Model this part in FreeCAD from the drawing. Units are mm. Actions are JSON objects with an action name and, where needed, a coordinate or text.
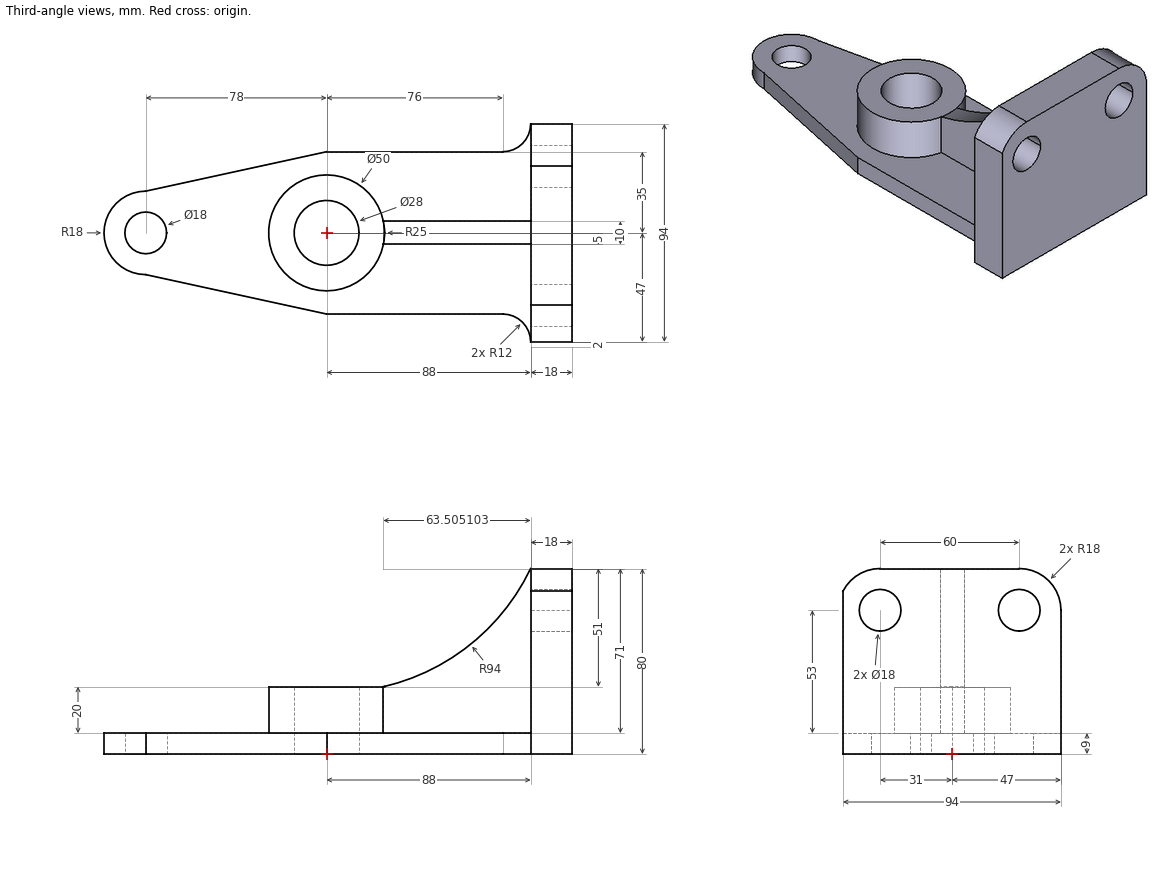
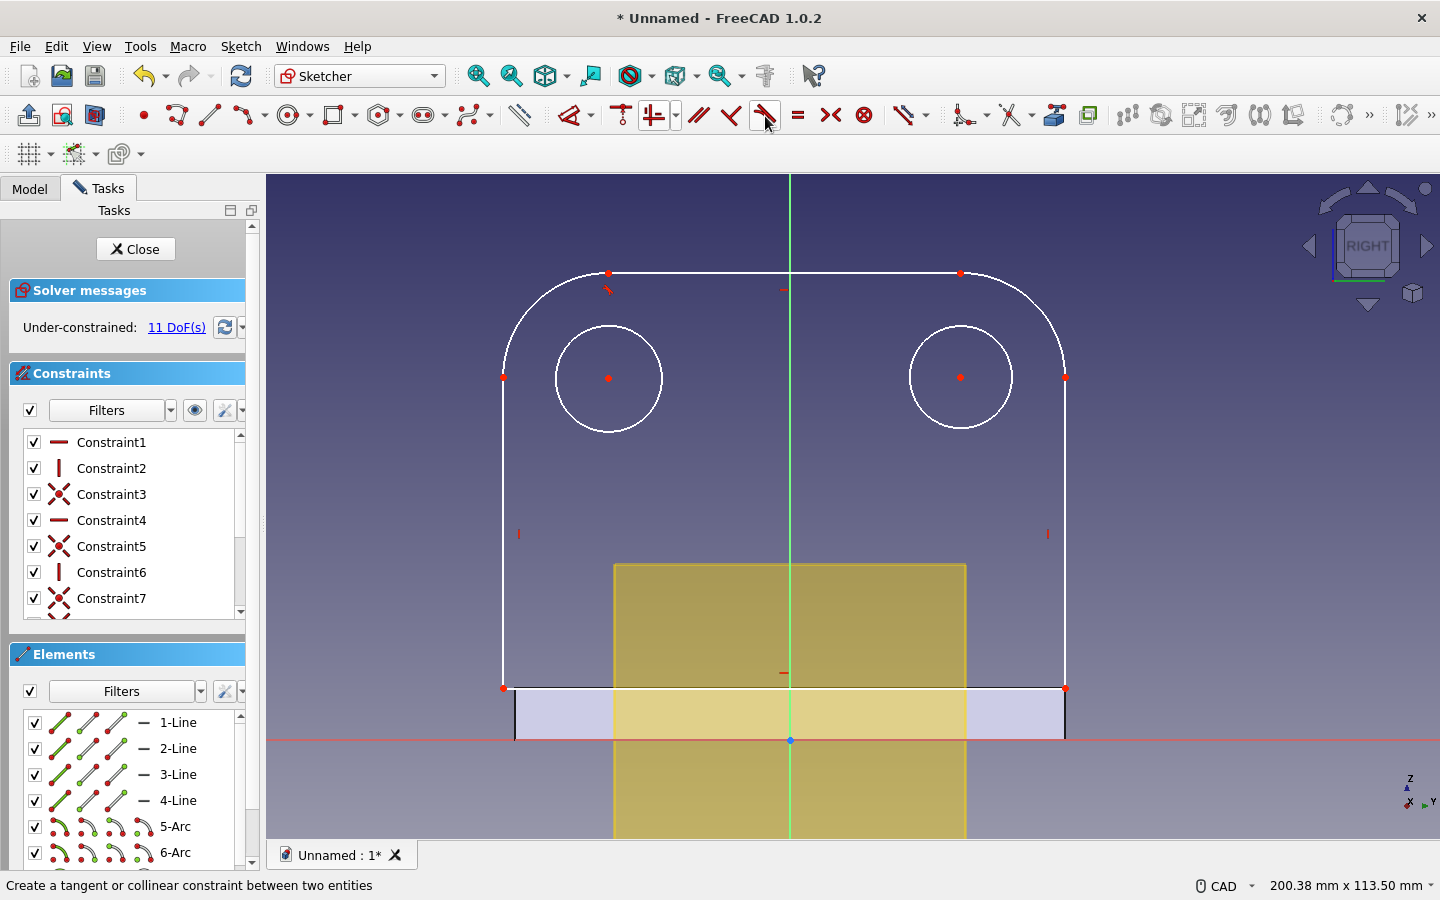
{"action": "left_click", "coordinate": [855, 273]}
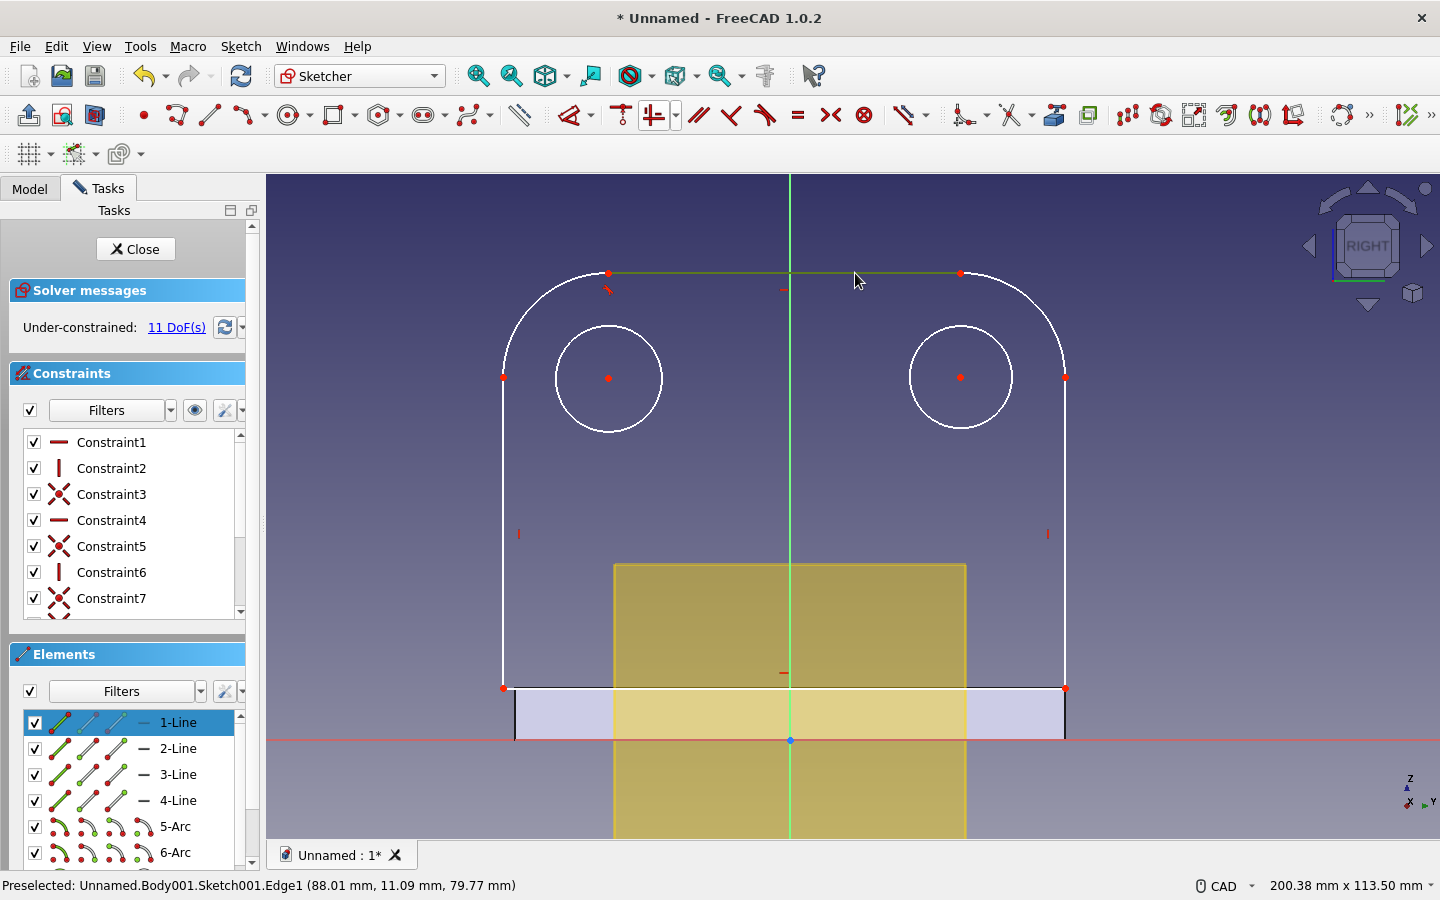
{"action": "left_click", "coordinate": [1054, 330]}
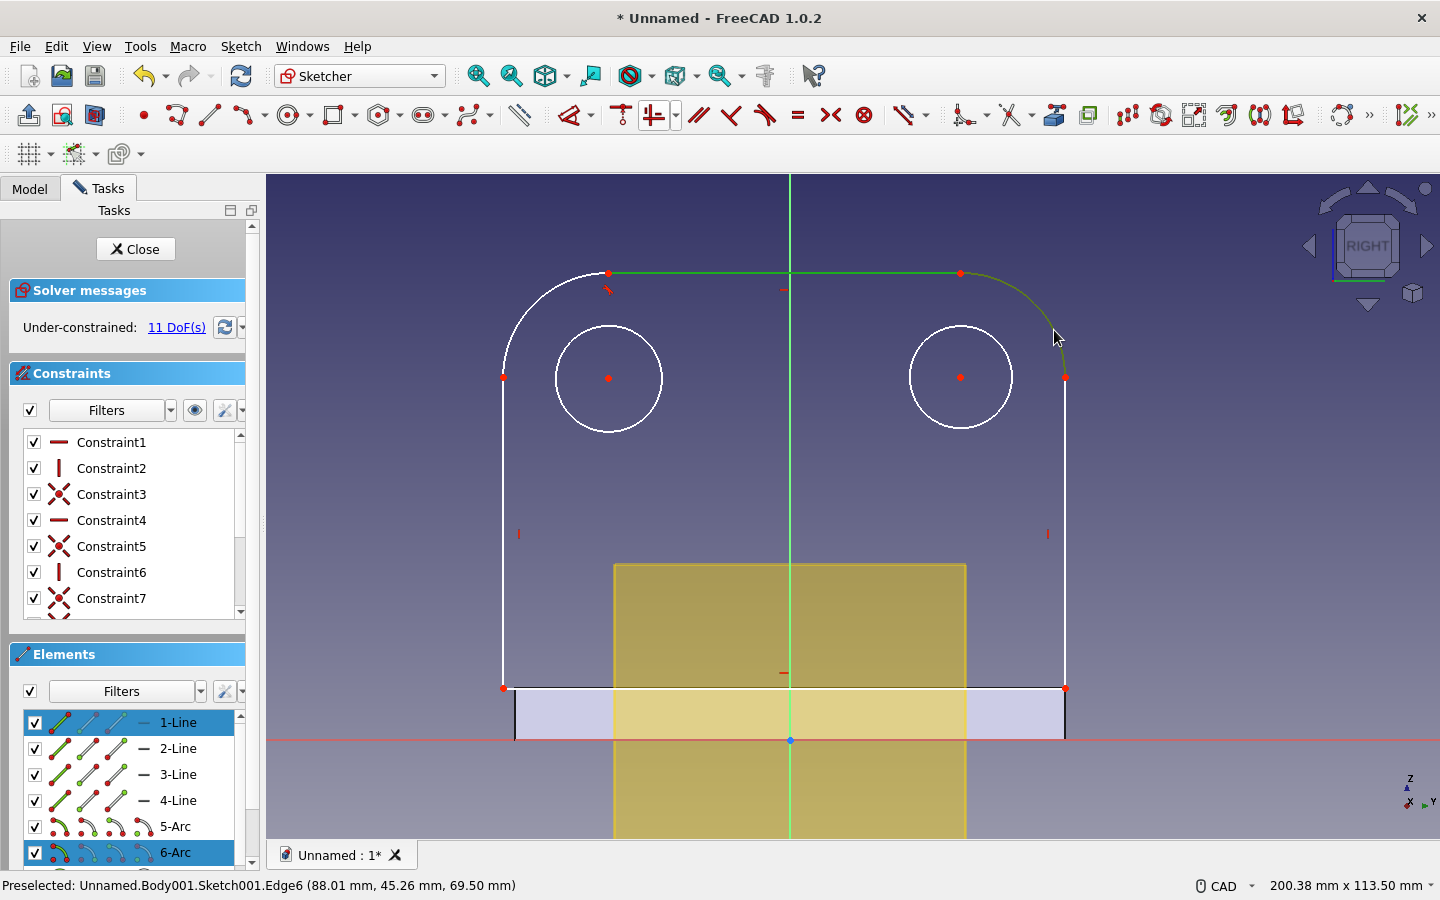
{"action": "left_click", "coordinate": [765, 116]}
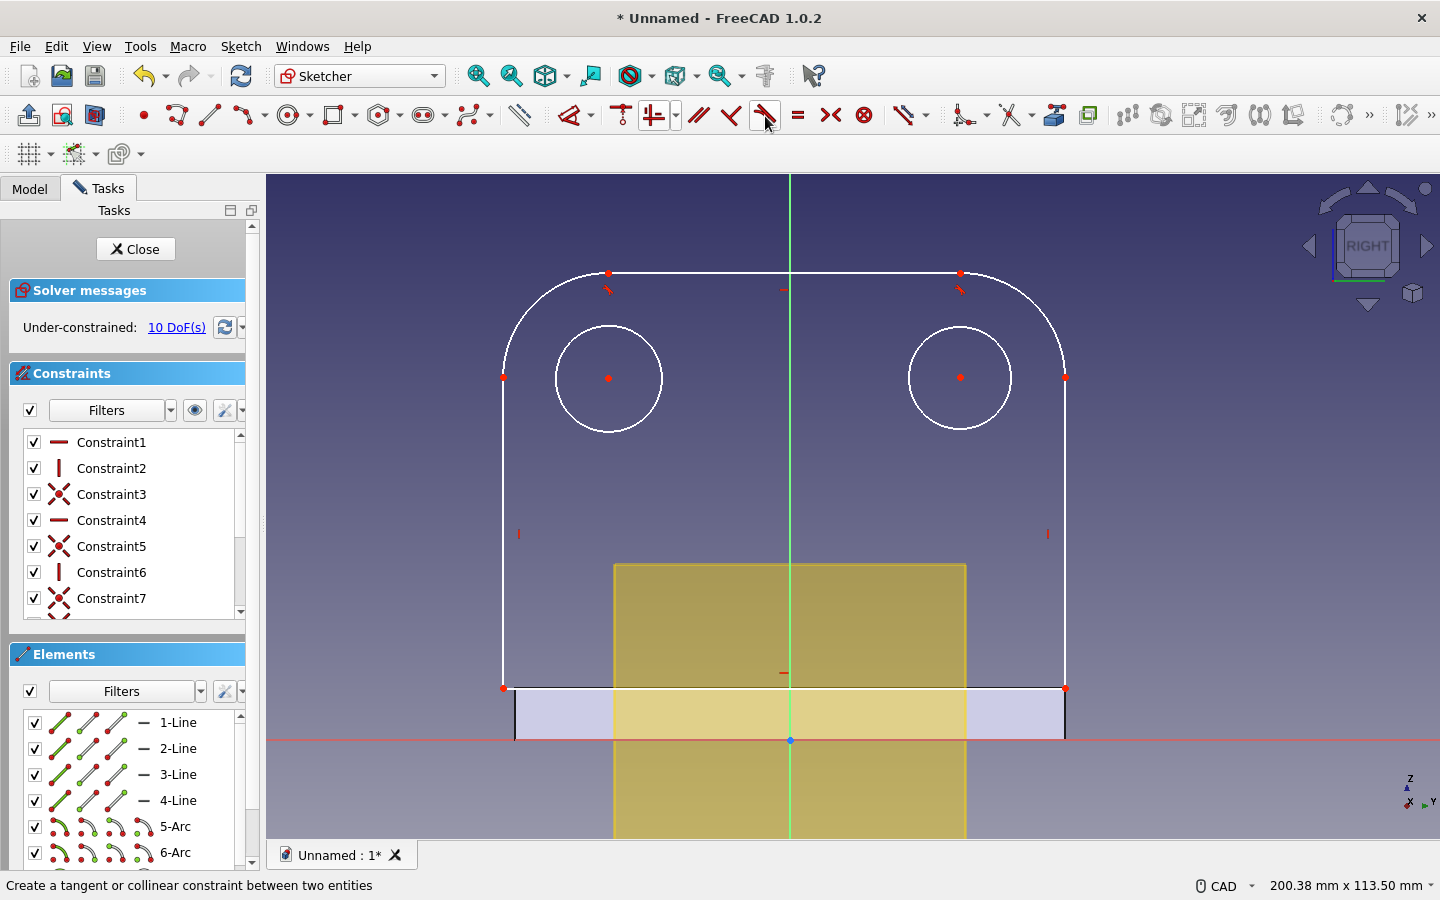
{"action": "left_click", "coordinate": [503, 471]}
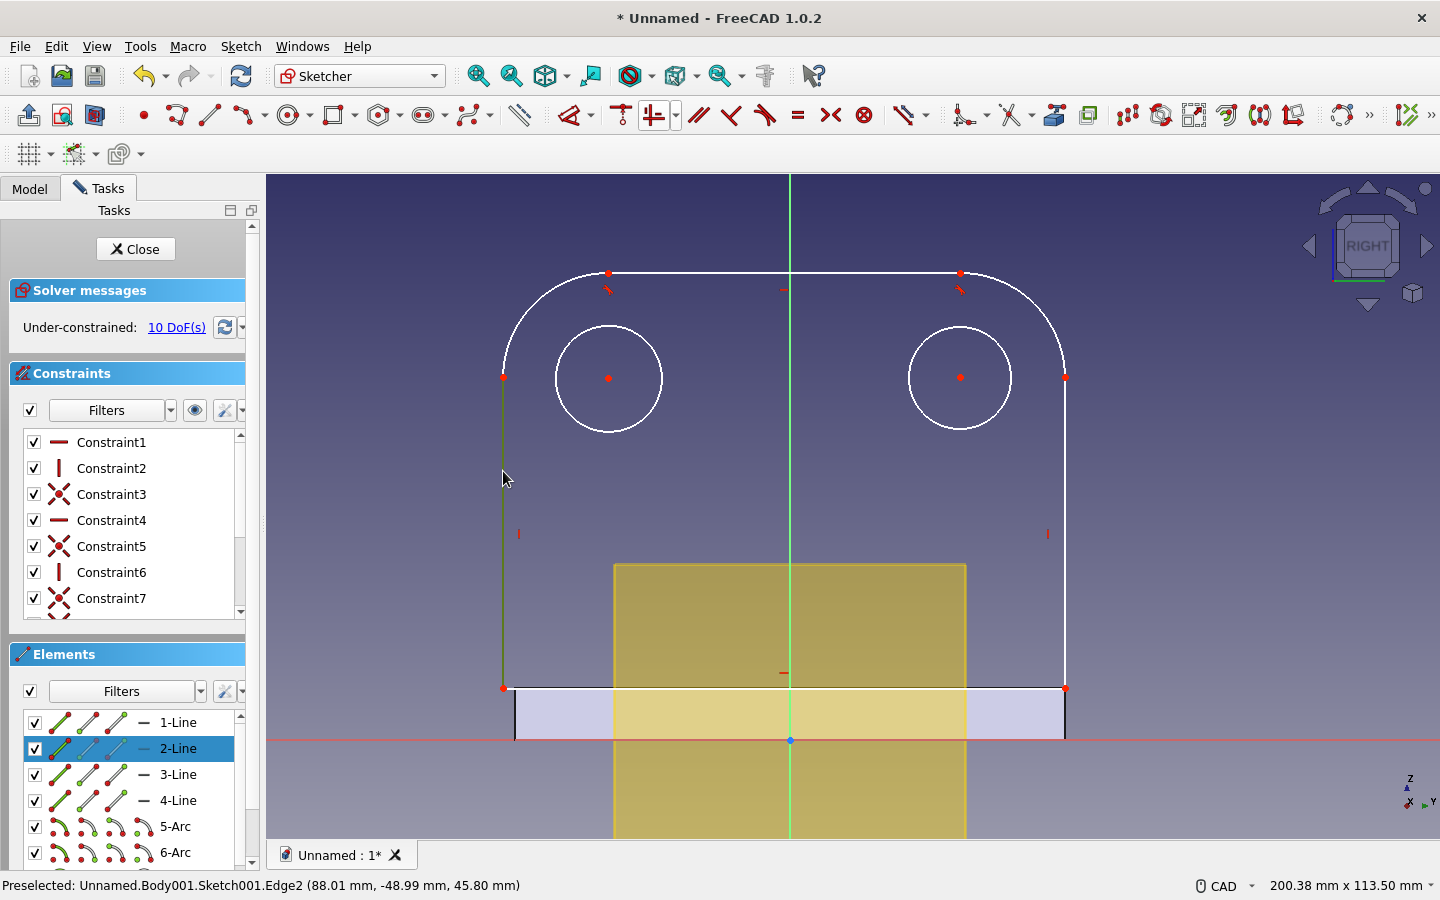
{"action": "left_click", "coordinate": [561, 284]}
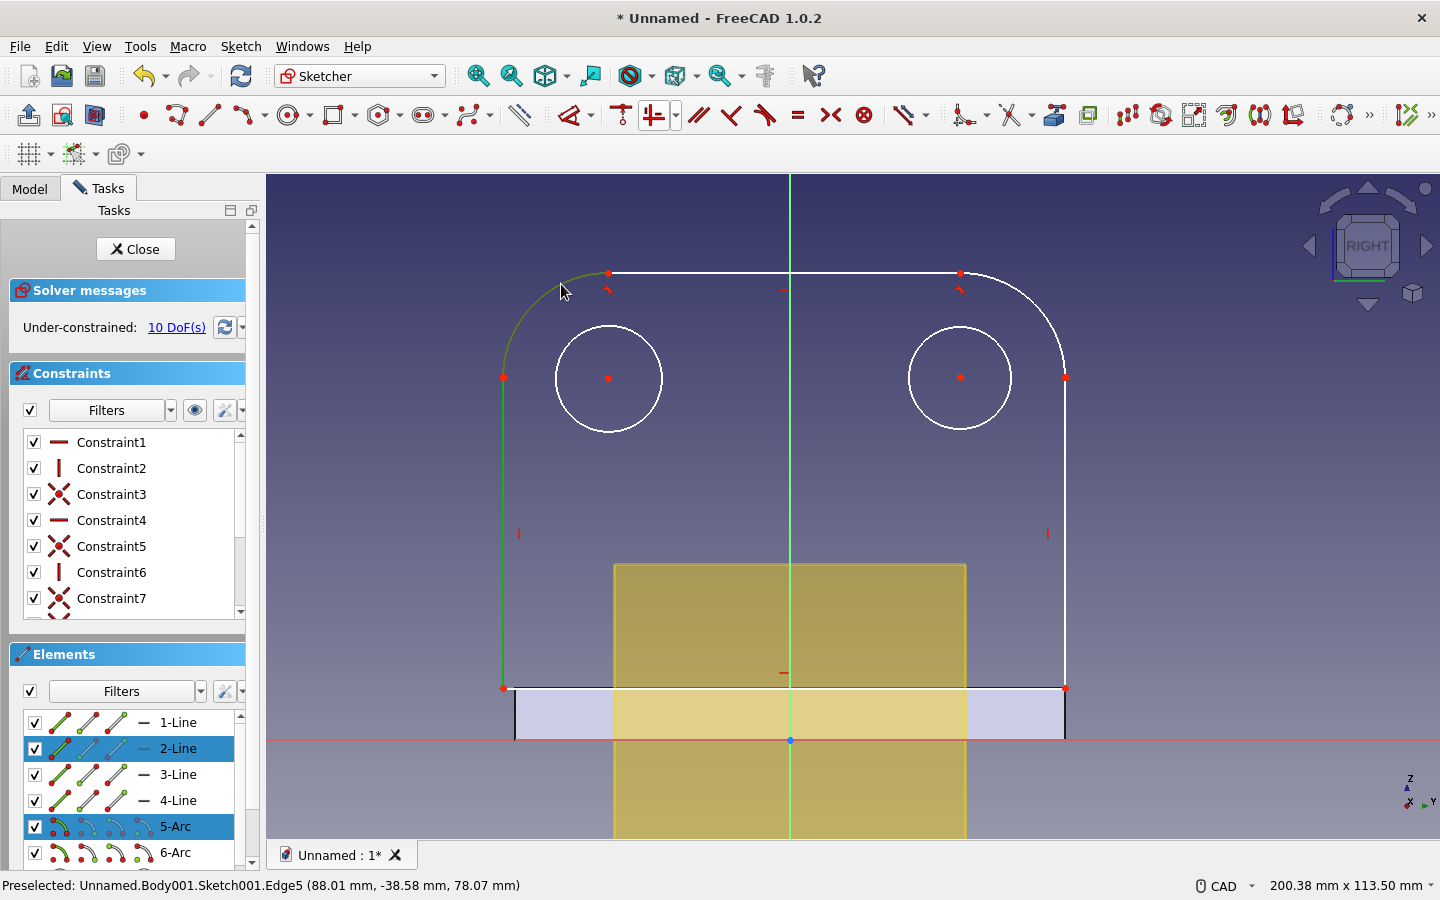
{"action": "key", "text": "t"}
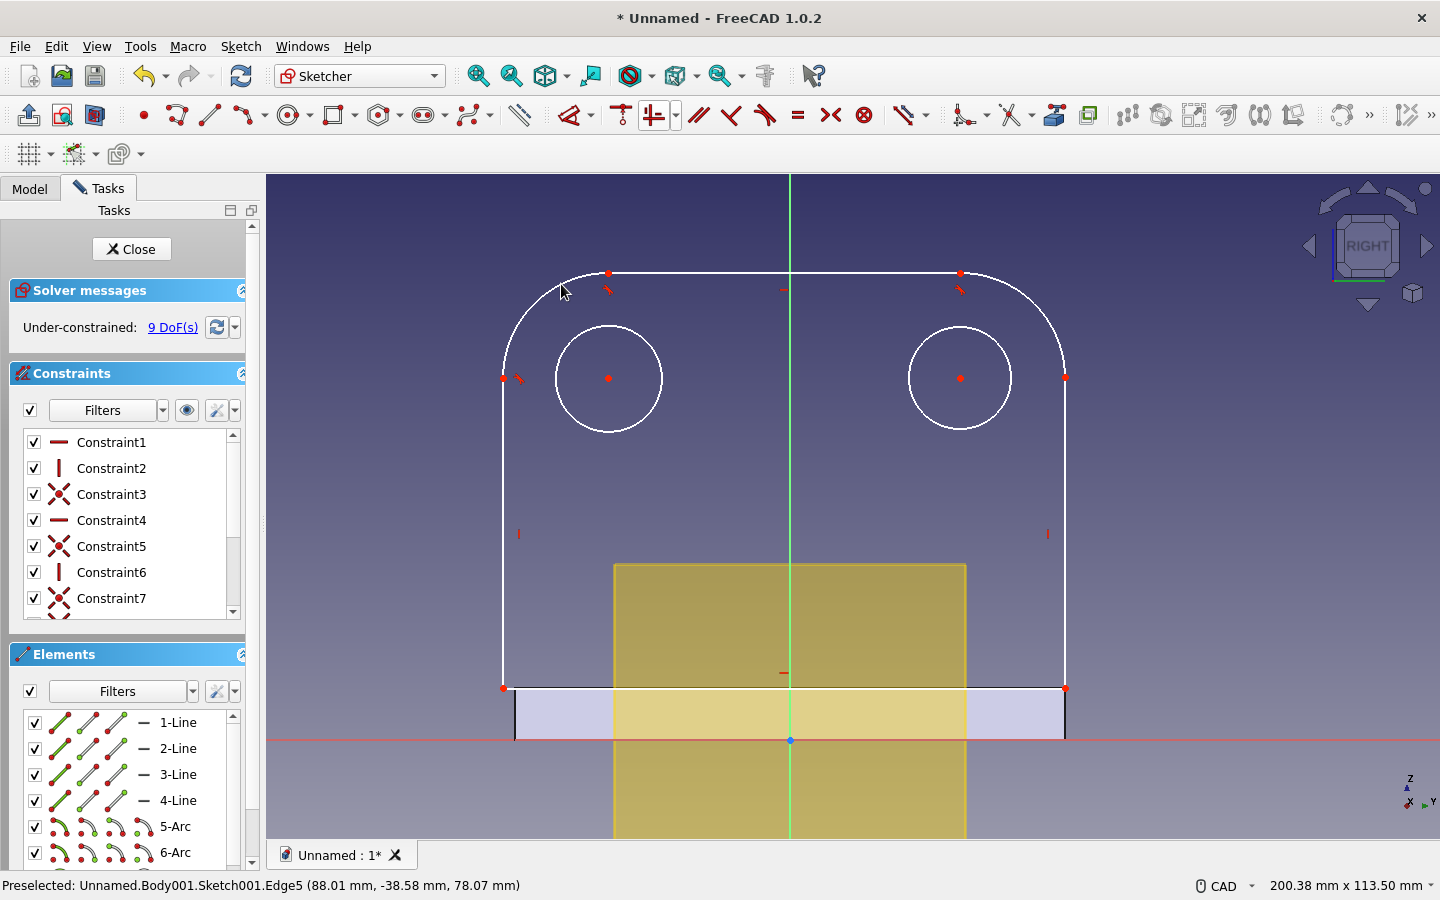
{"action": "left_click", "coordinate": [1065, 596]}